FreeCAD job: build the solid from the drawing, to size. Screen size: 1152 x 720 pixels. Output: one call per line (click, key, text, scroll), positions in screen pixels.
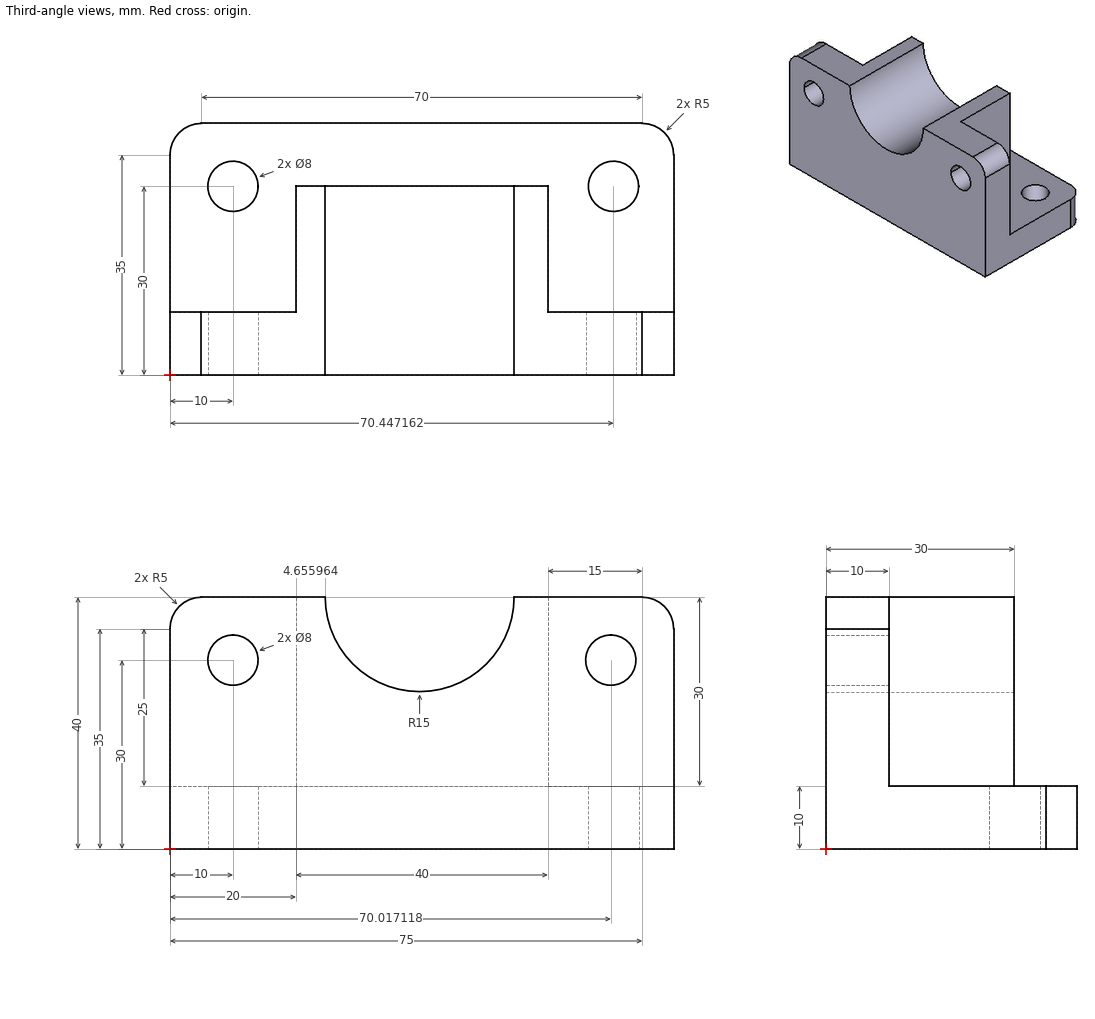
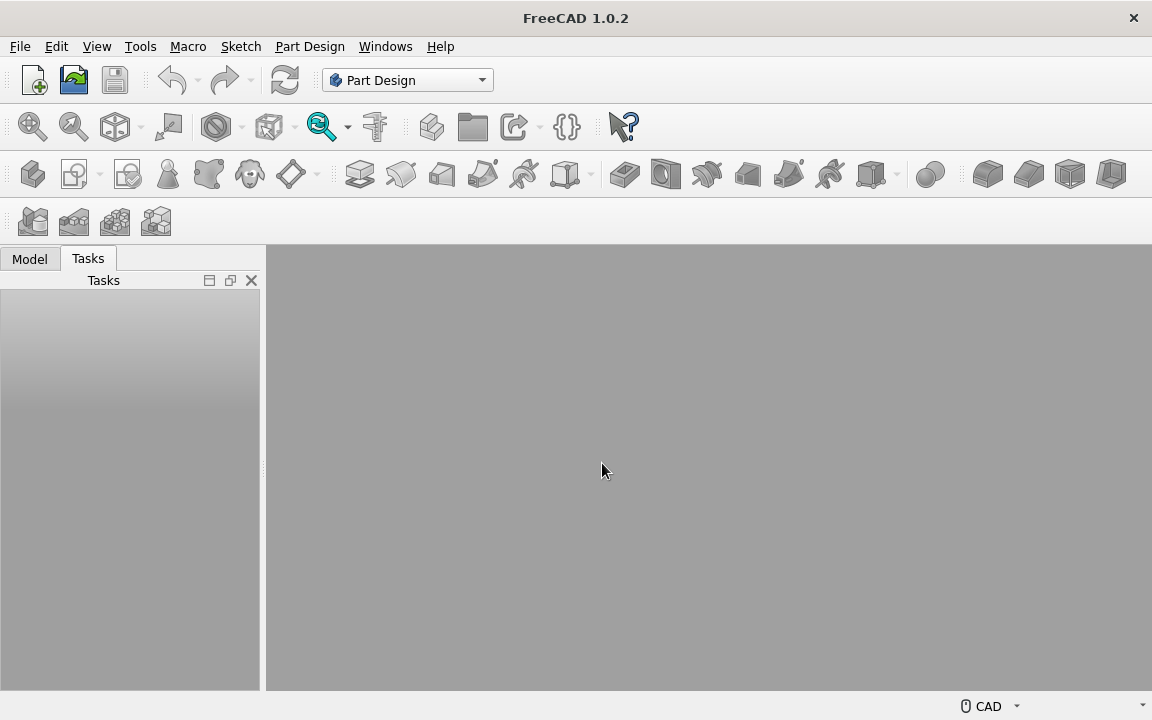
click(33, 80)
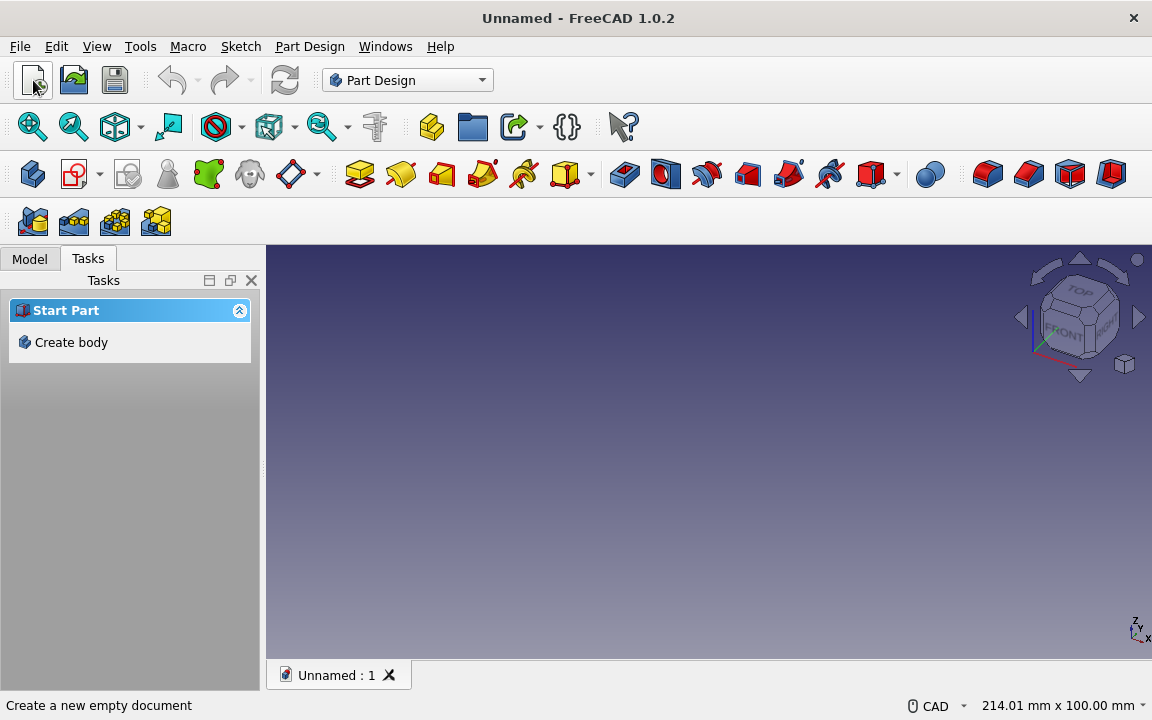
click(74, 174)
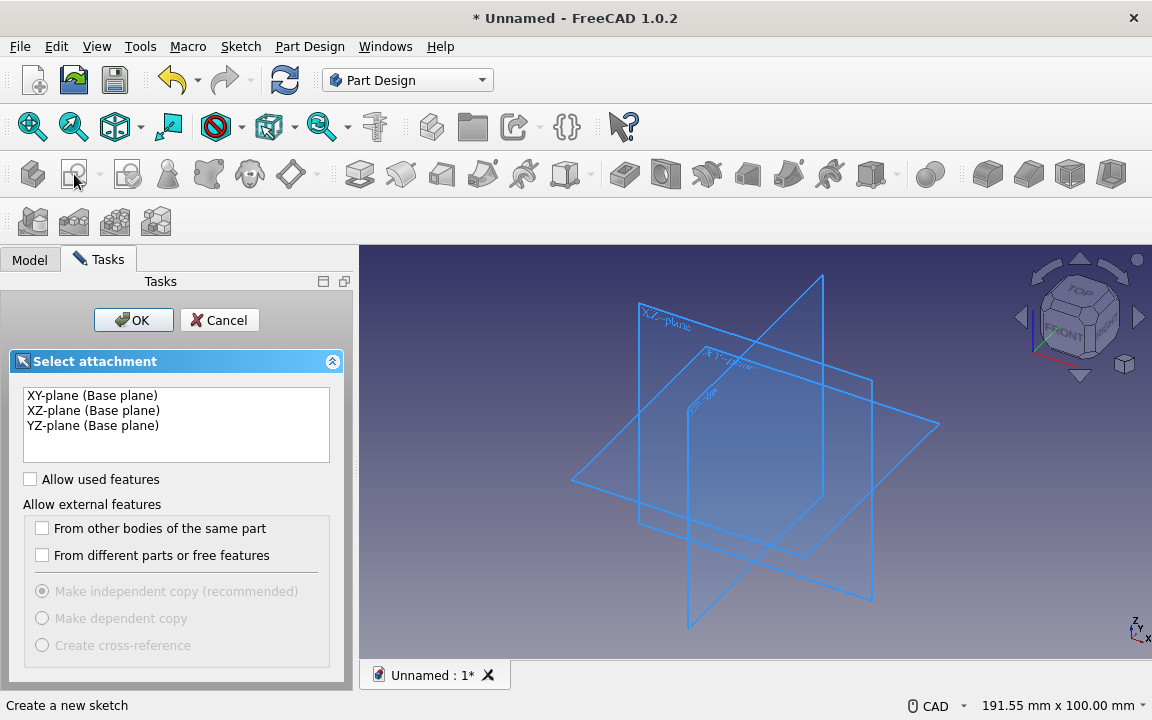
click(84, 396)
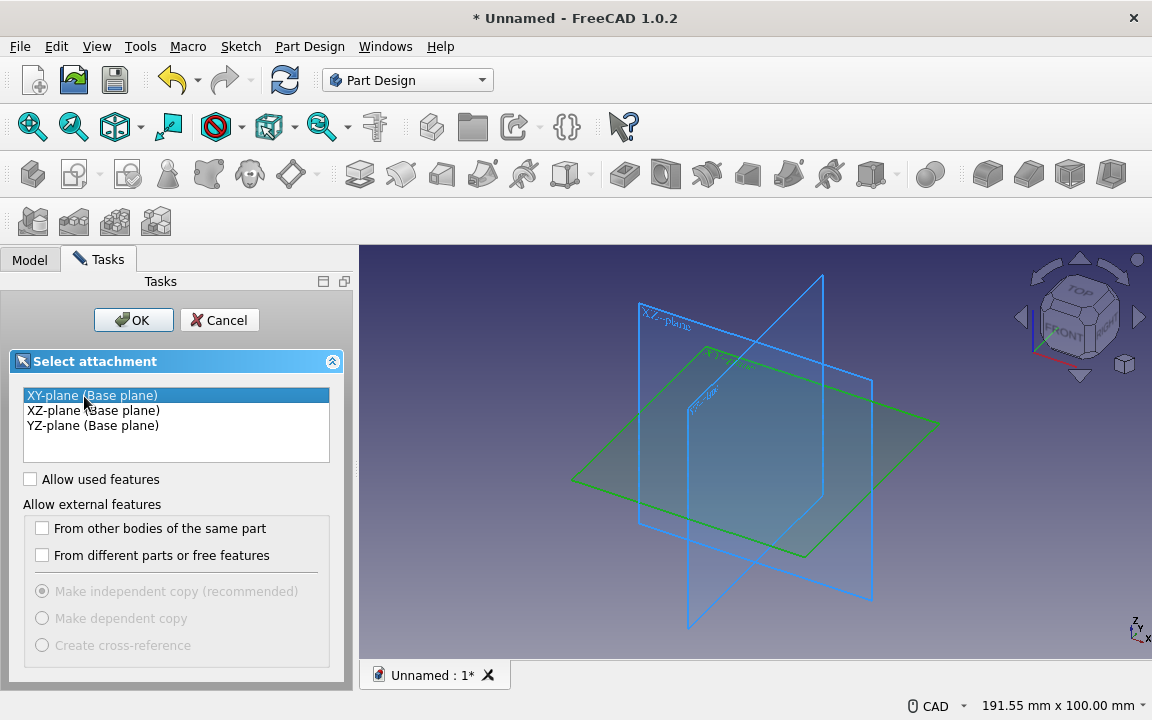
click(134, 320)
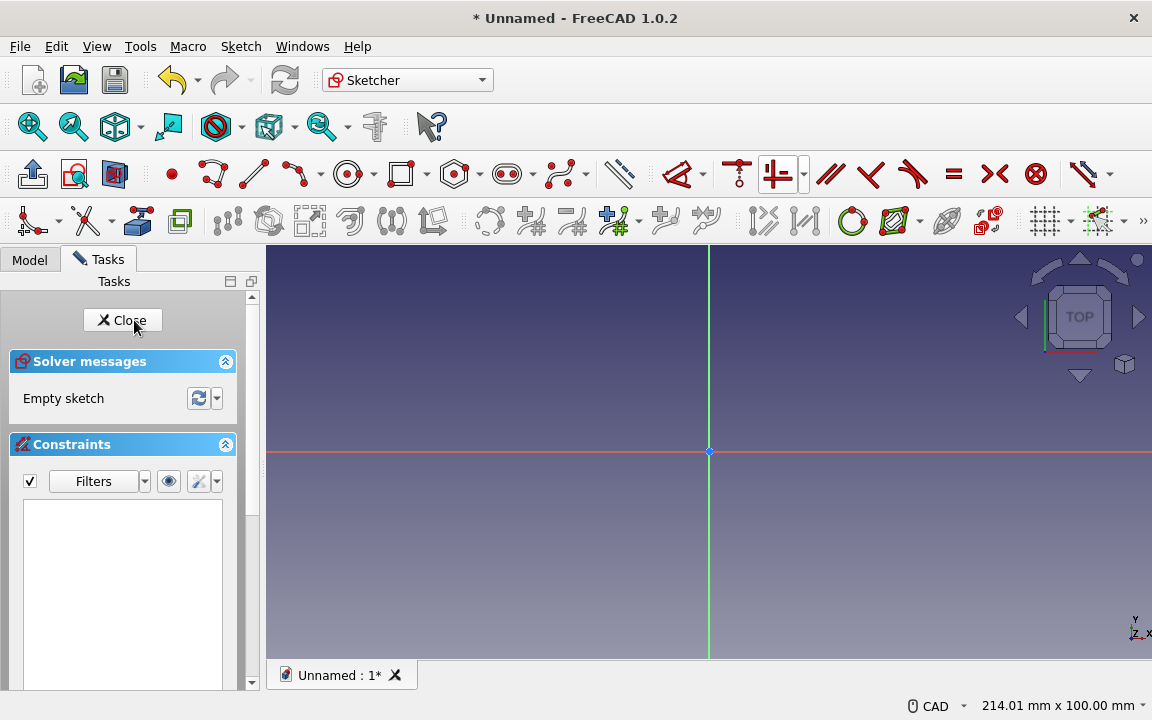
scroll(294, 631, down, 1)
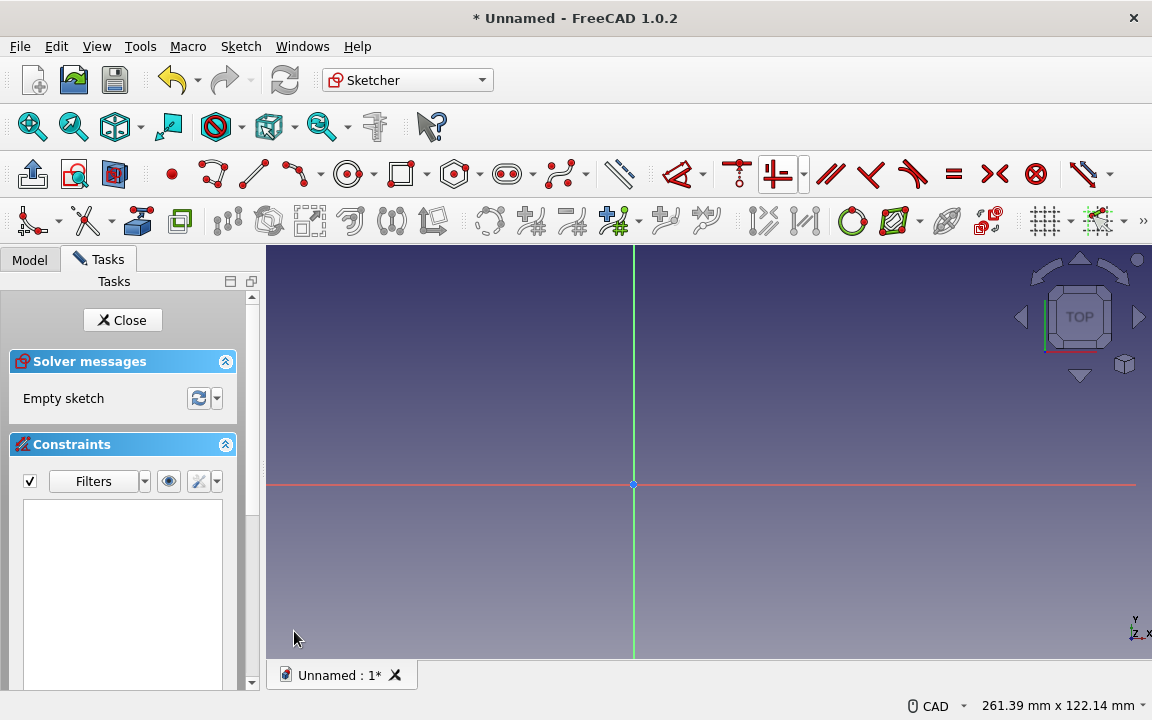
scroll(926, 374, up, 3)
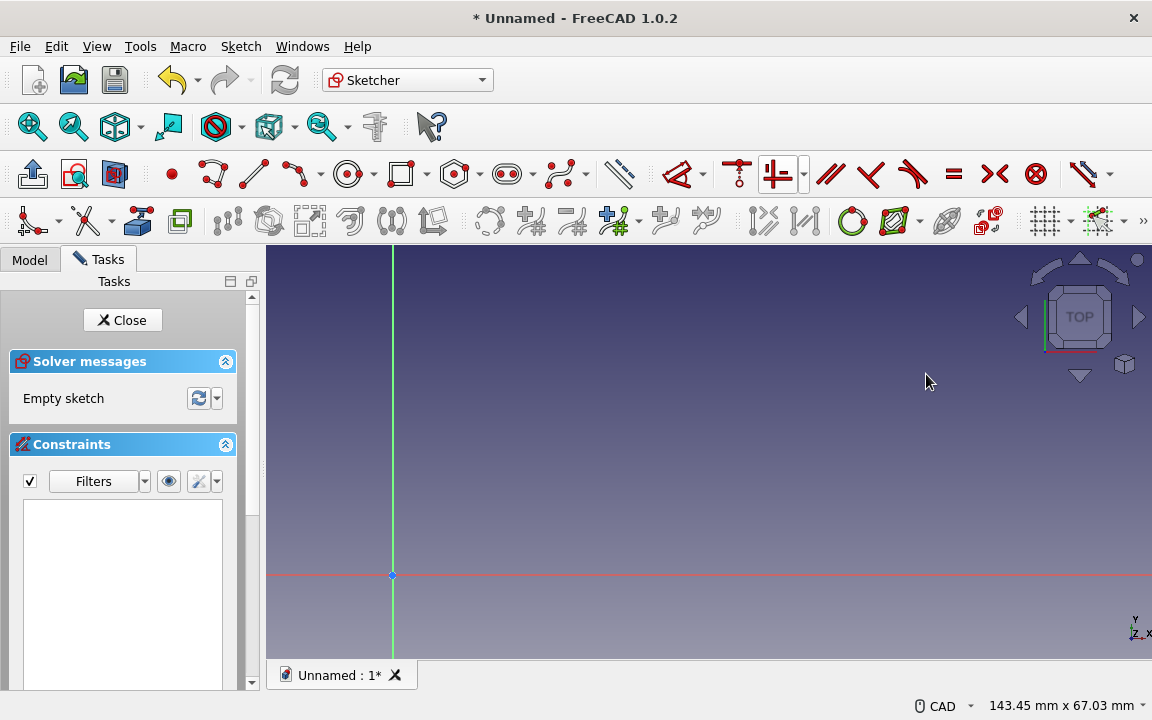
key(g)
key(l)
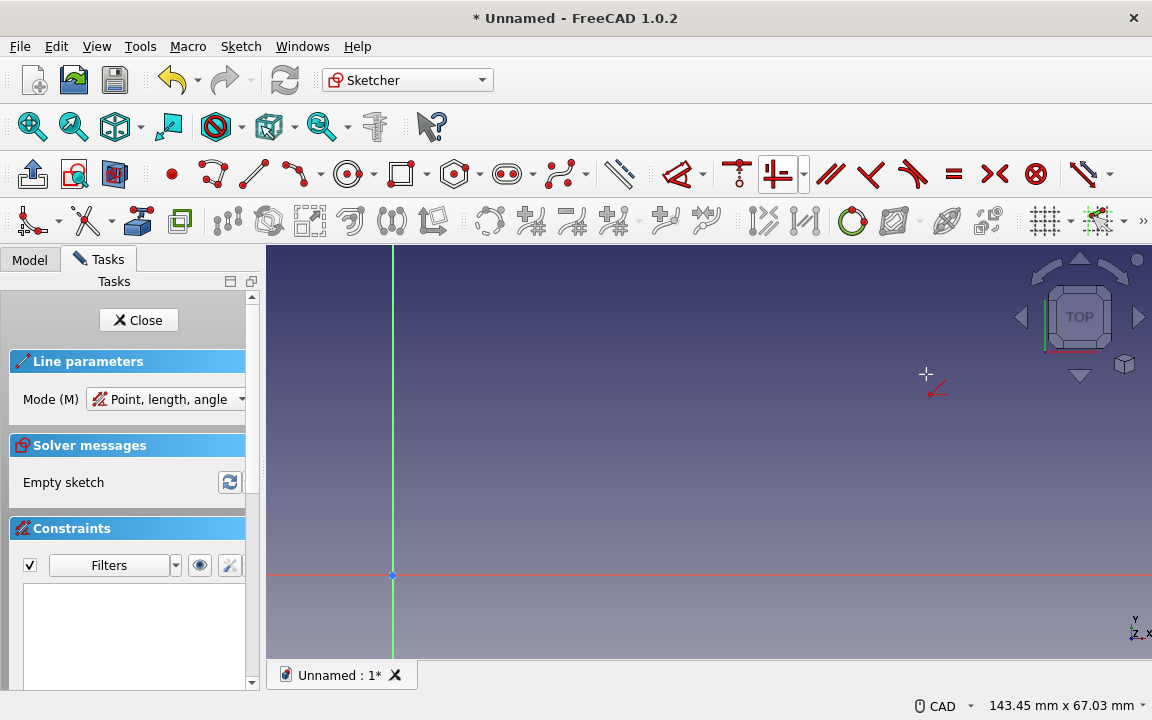
click(856, 328)
click(424, 328)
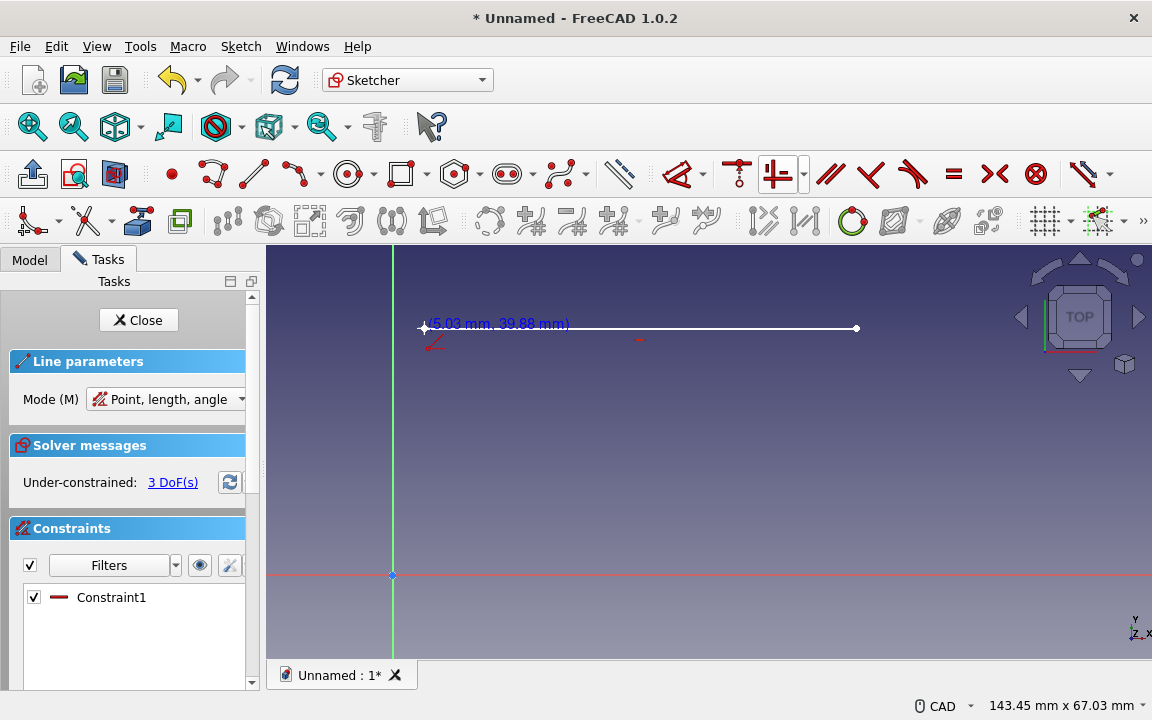
key(g)
key(m)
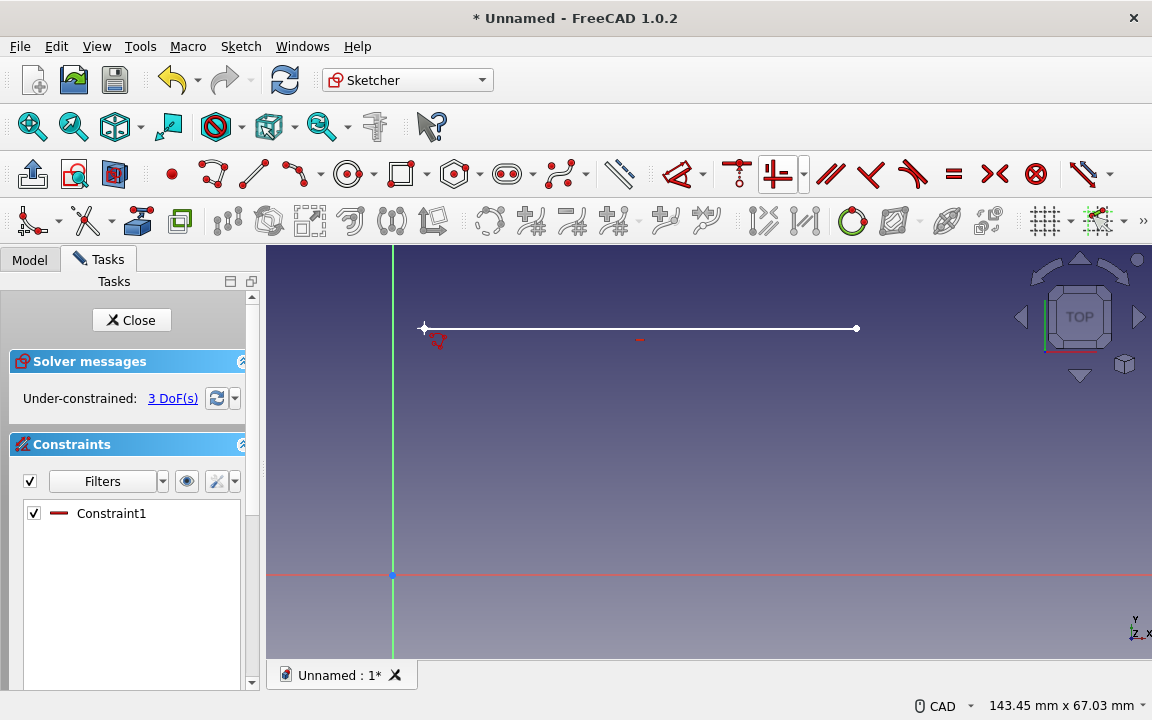
click(393, 359)
click(393, 575)
click(887, 566)
click(887, 359)
right_click(887, 359)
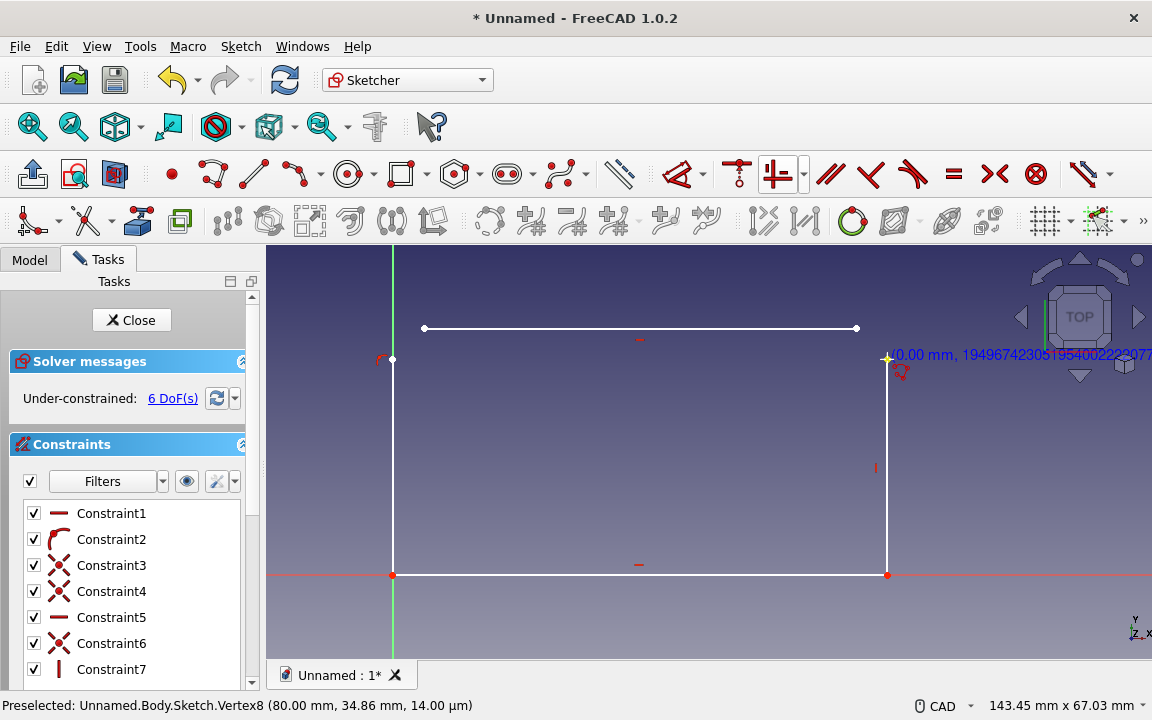
click(294, 174)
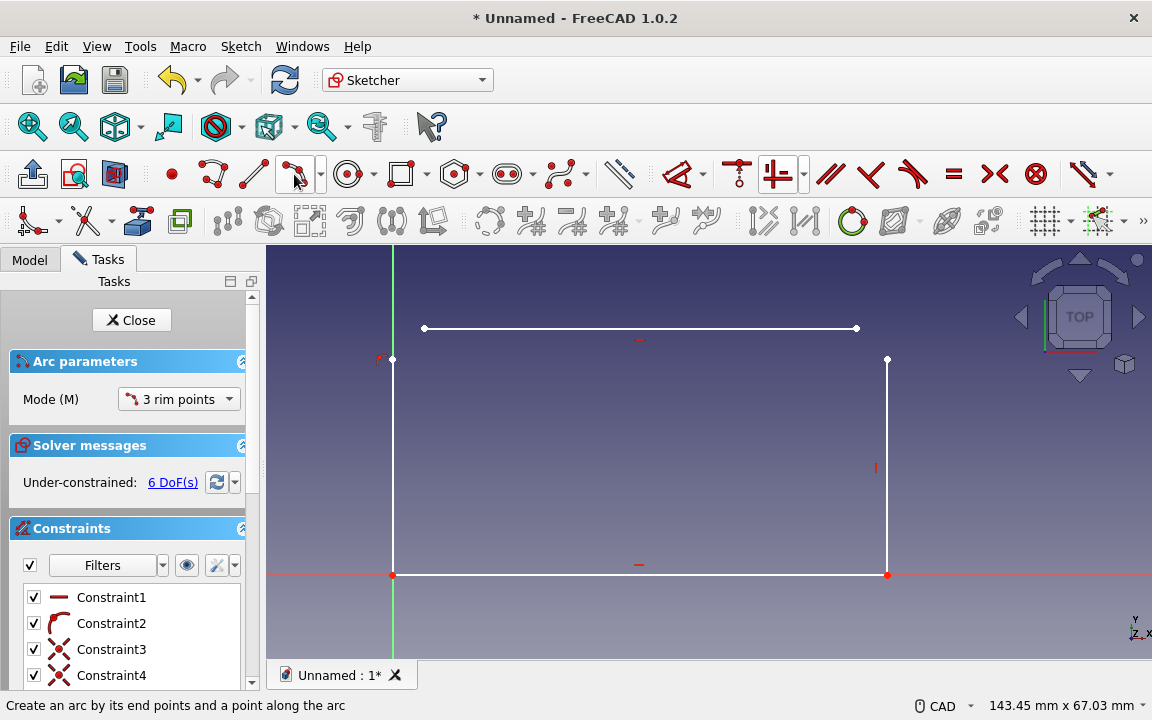
click(424, 329)
click(393, 360)